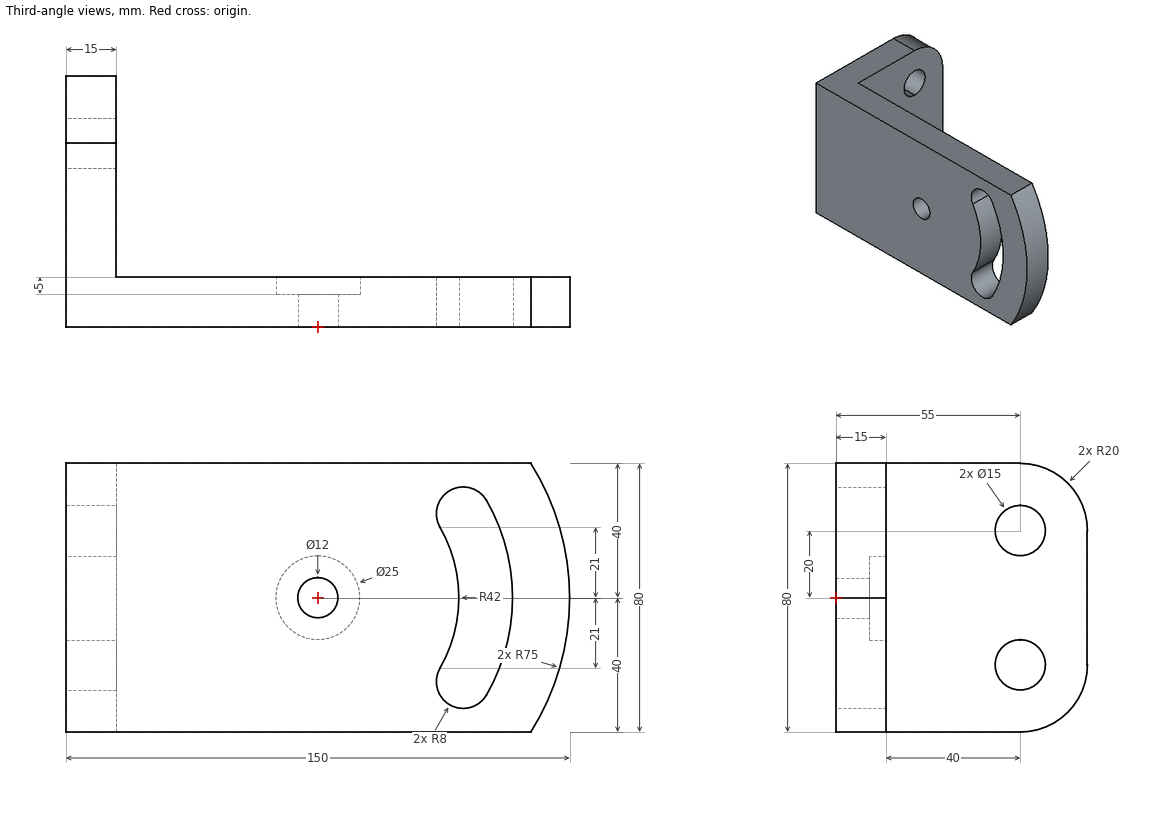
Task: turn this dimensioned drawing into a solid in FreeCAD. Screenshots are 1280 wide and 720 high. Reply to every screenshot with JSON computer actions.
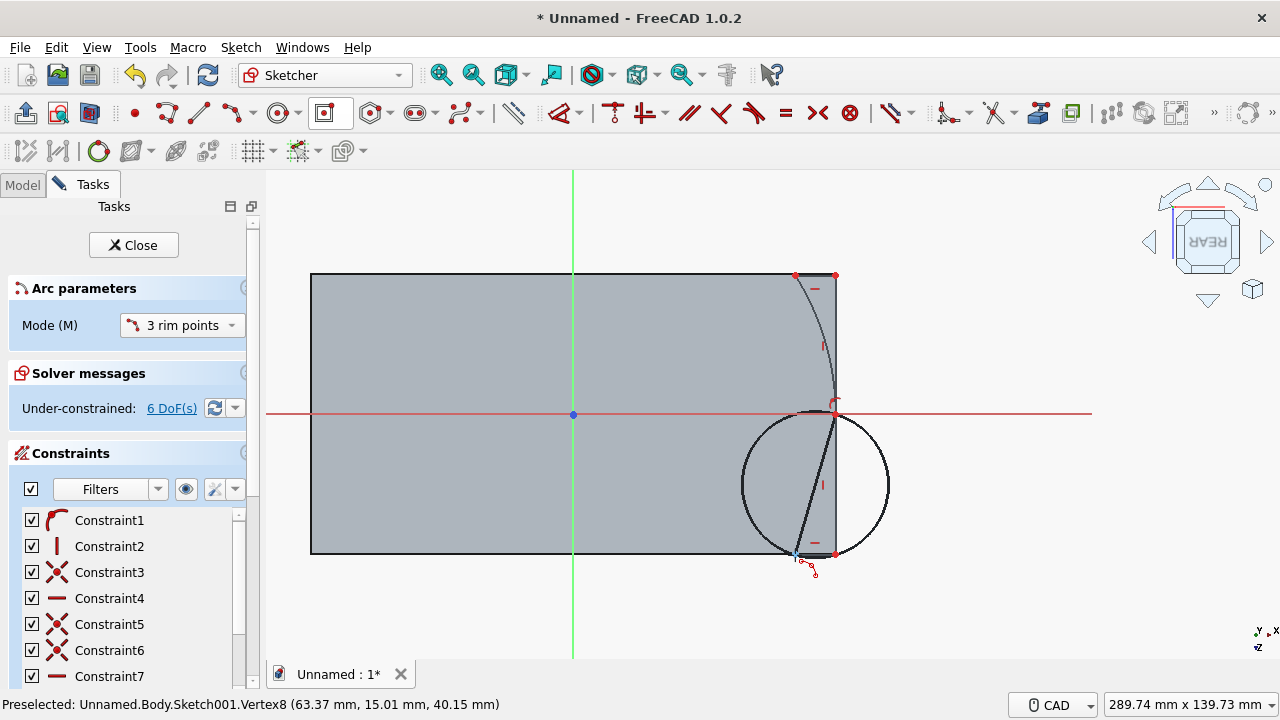
{"action": "scroll", "coordinate": [825, 487], "scroll_direction": "up", "scroll_amount": 3}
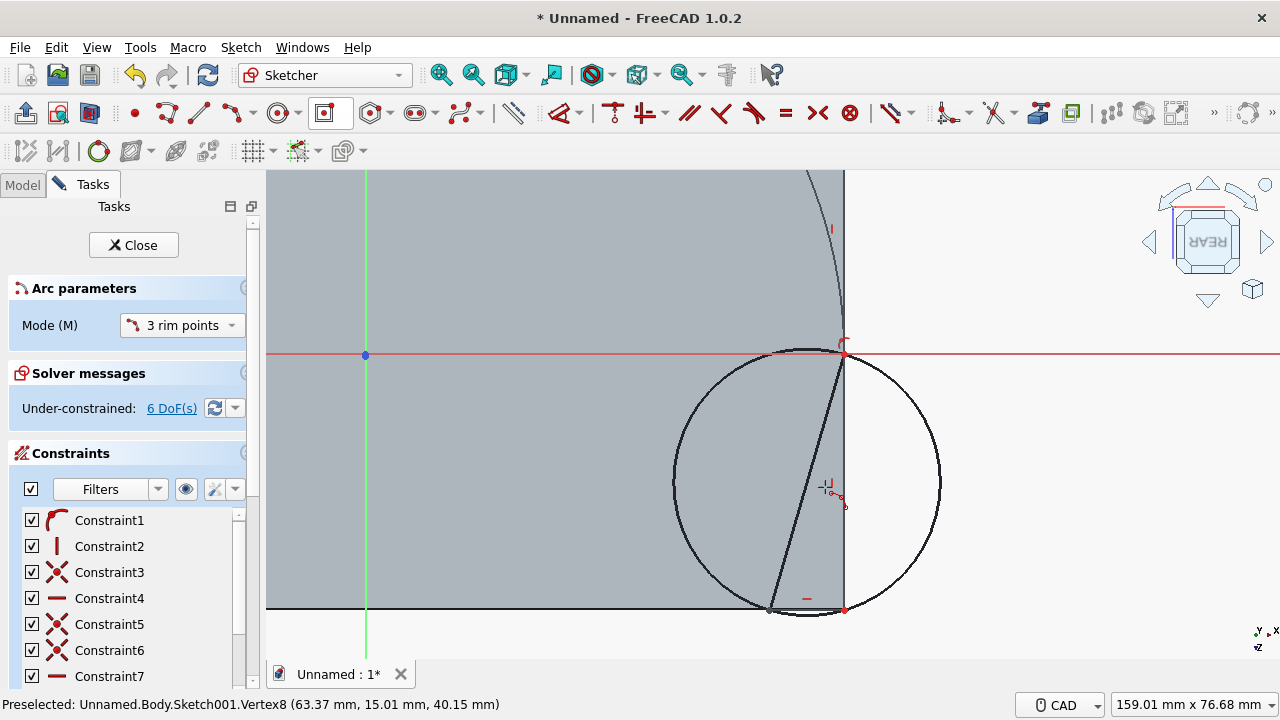
{"action": "left_click", "coordinate": [825, 487]}
{"action": "key", "text": "Escape"}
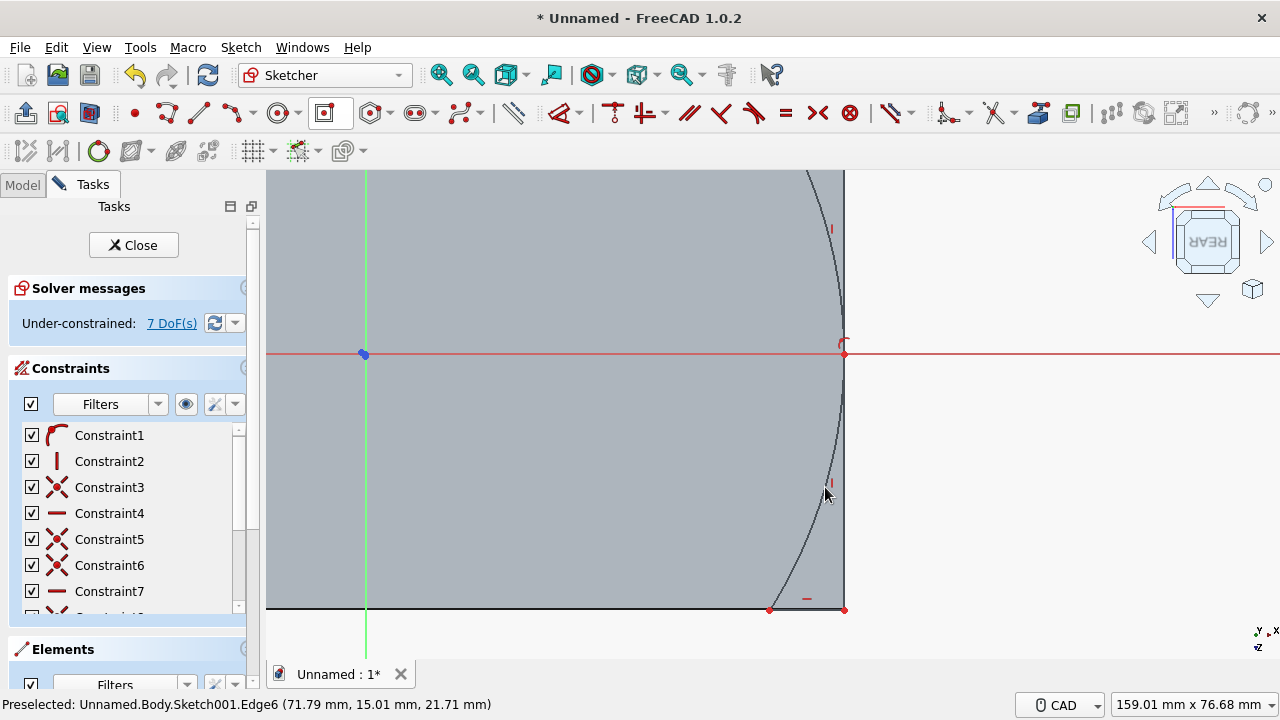
{"action": "left_click", "coordinate": [825, 223]}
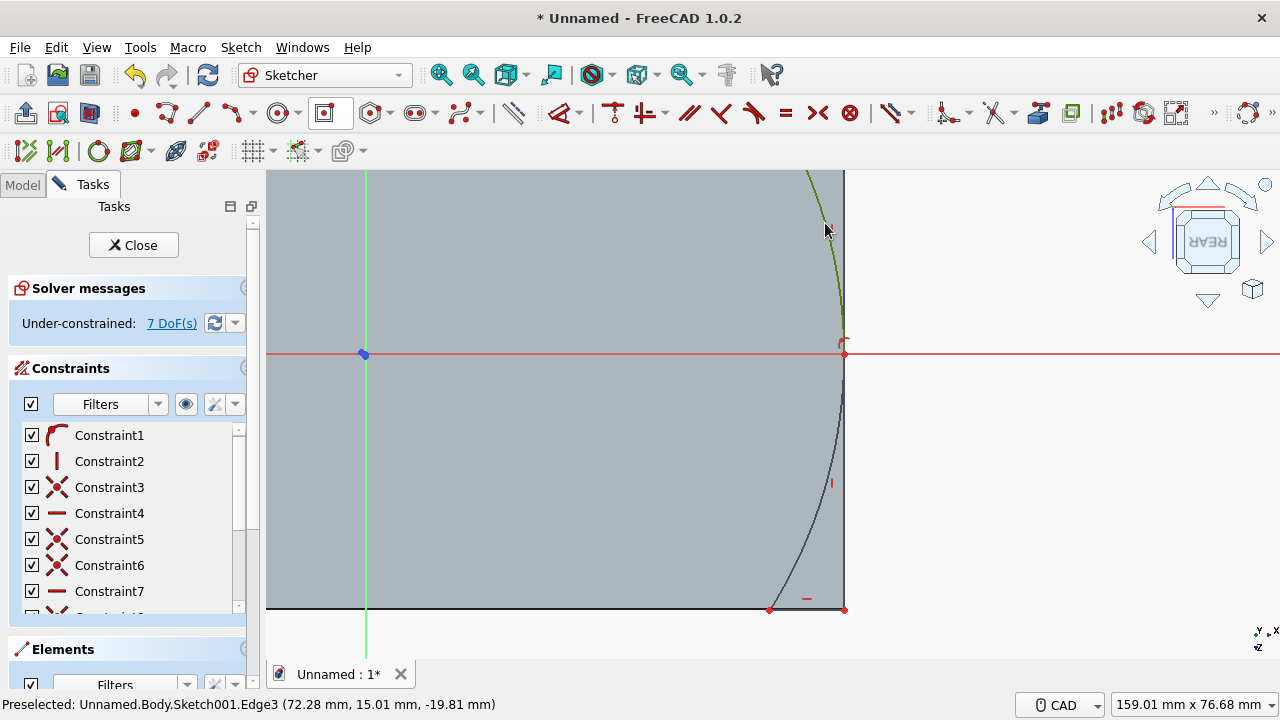
{"action": "left_click", "coordinate": [807, 539]}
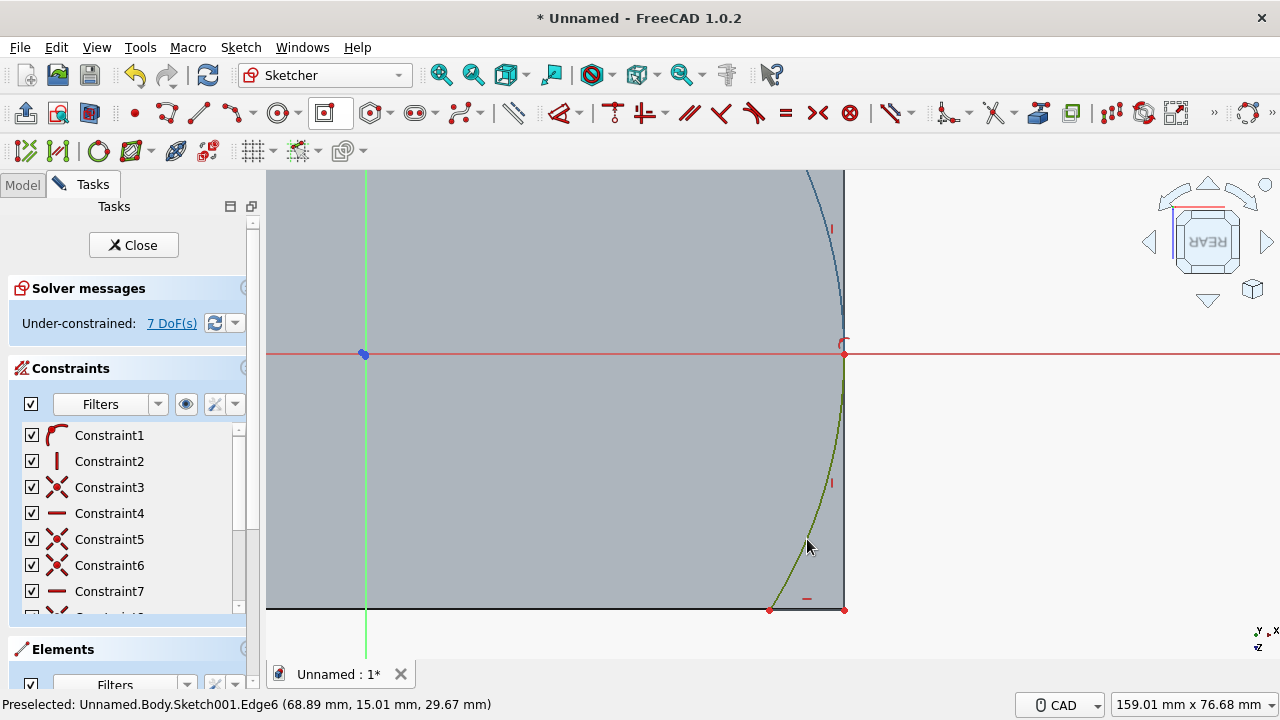
{"action": "left_click", "coordinate": [614, 114]}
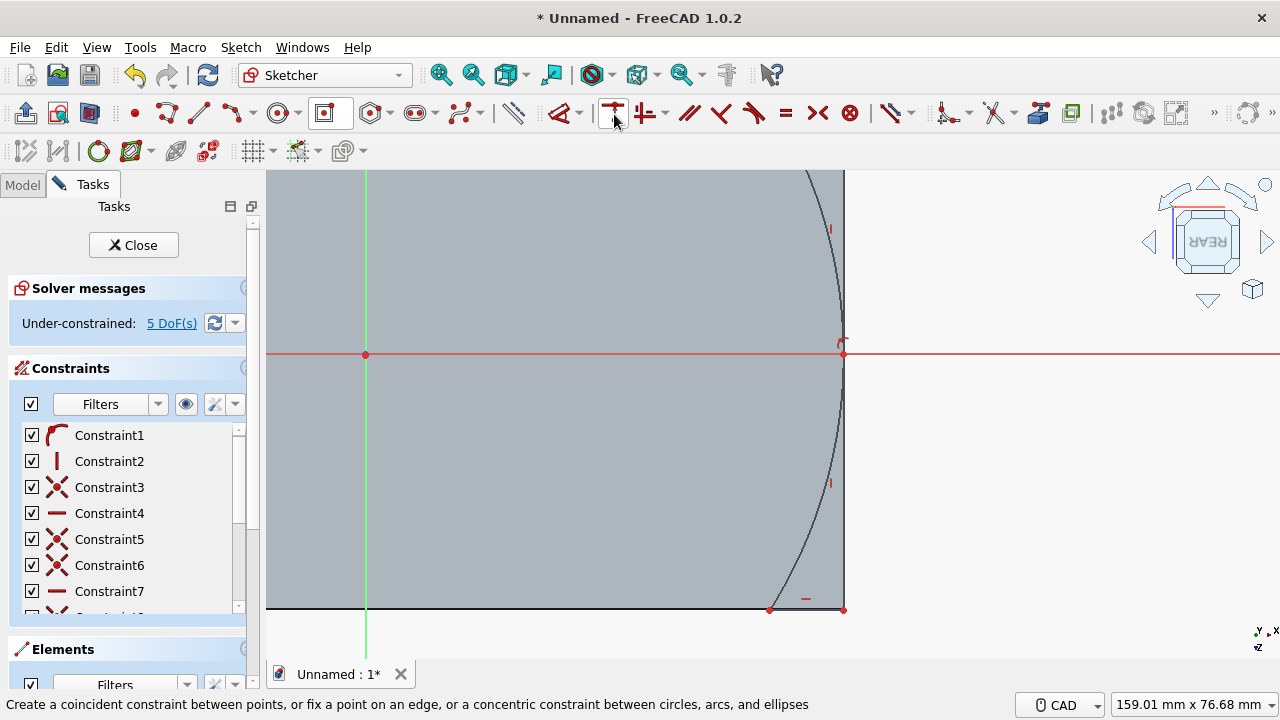
{"action": "left_click_drag", "start_coordinate": [356, 344], "coordinate": [376, 365]}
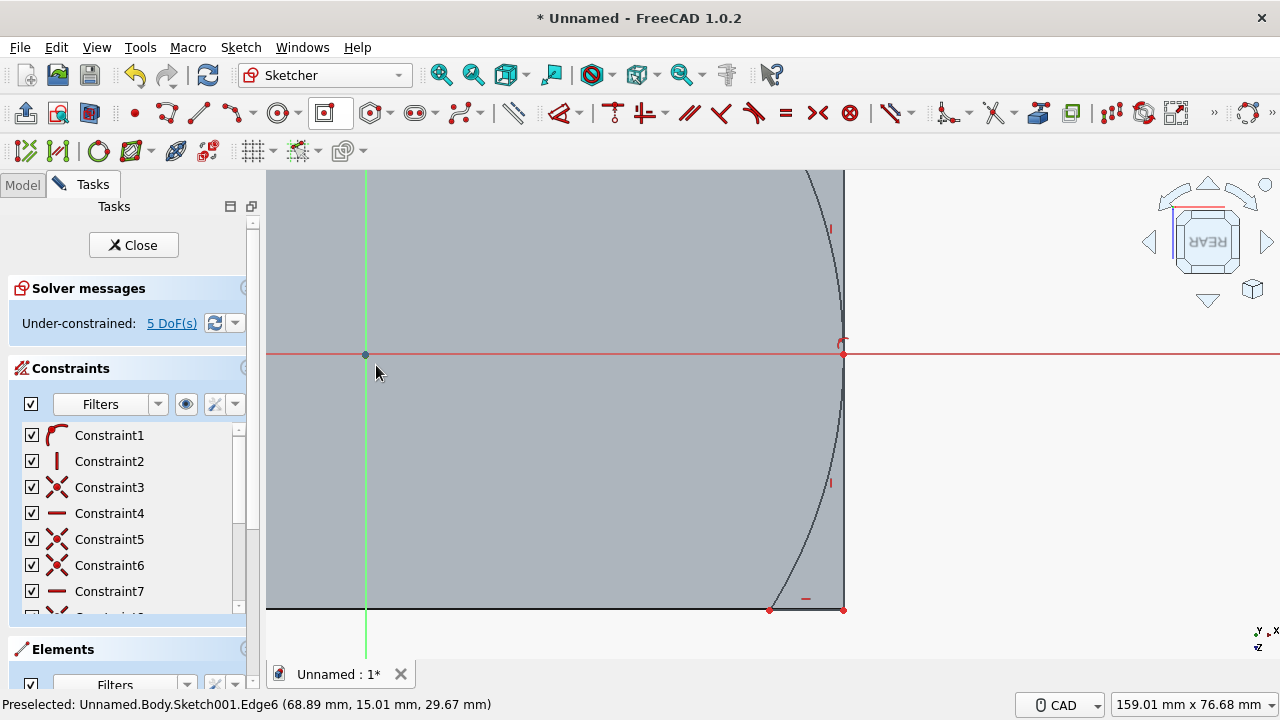
{"action": "left_click", "coordinate": [614, 114]}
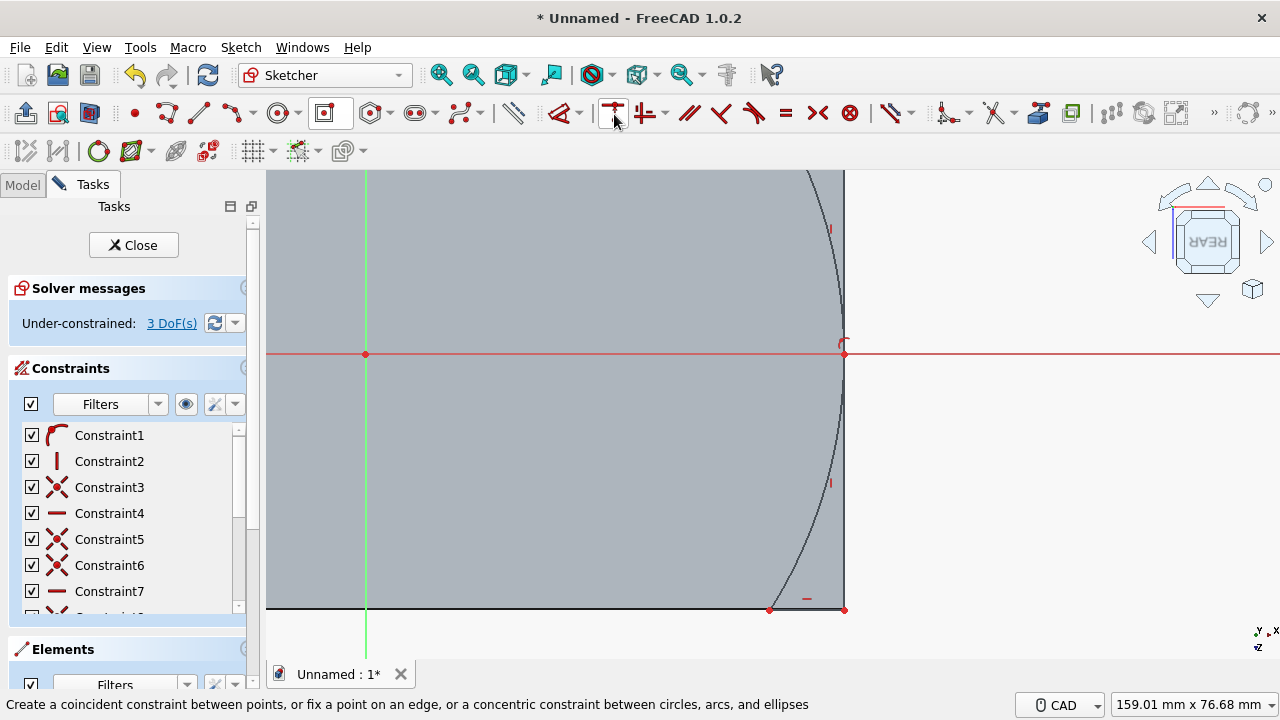
{"action": "left_click", "coordinate": [560, 114]}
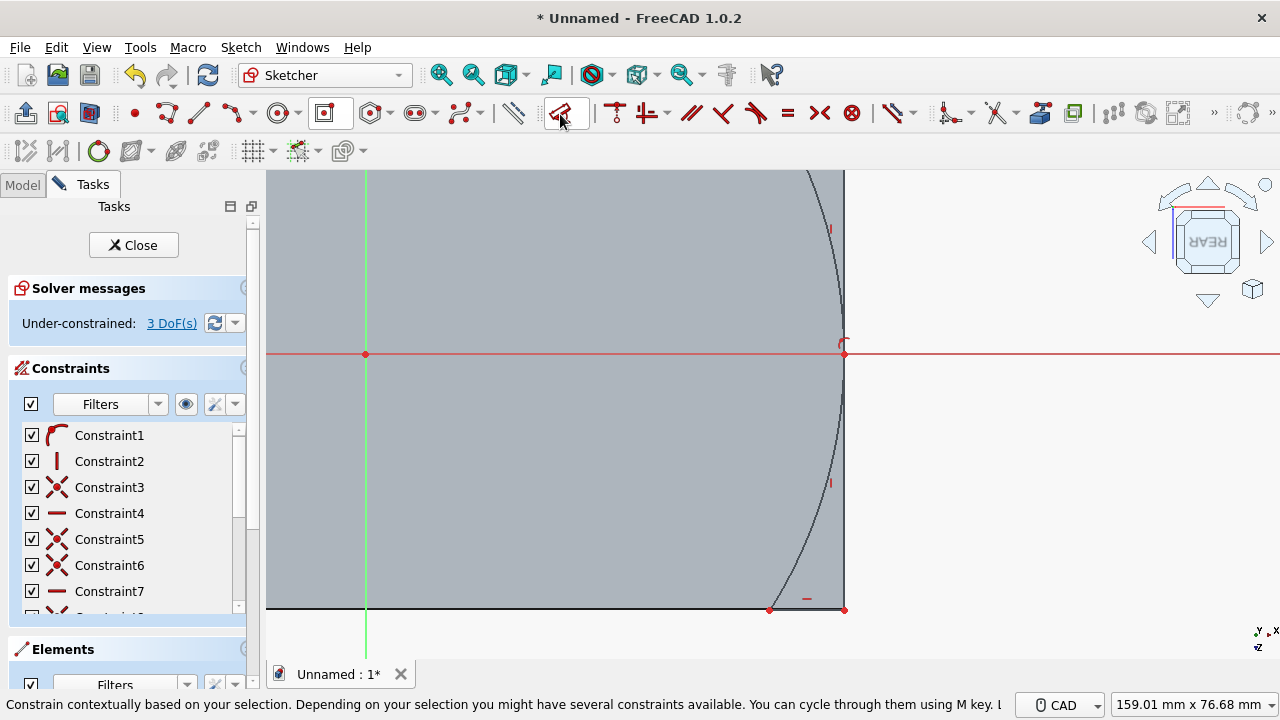
{"action": "left_click", "coordinate": [826, 223]}
{"action": "left_click", "coordinate": [864, 467]}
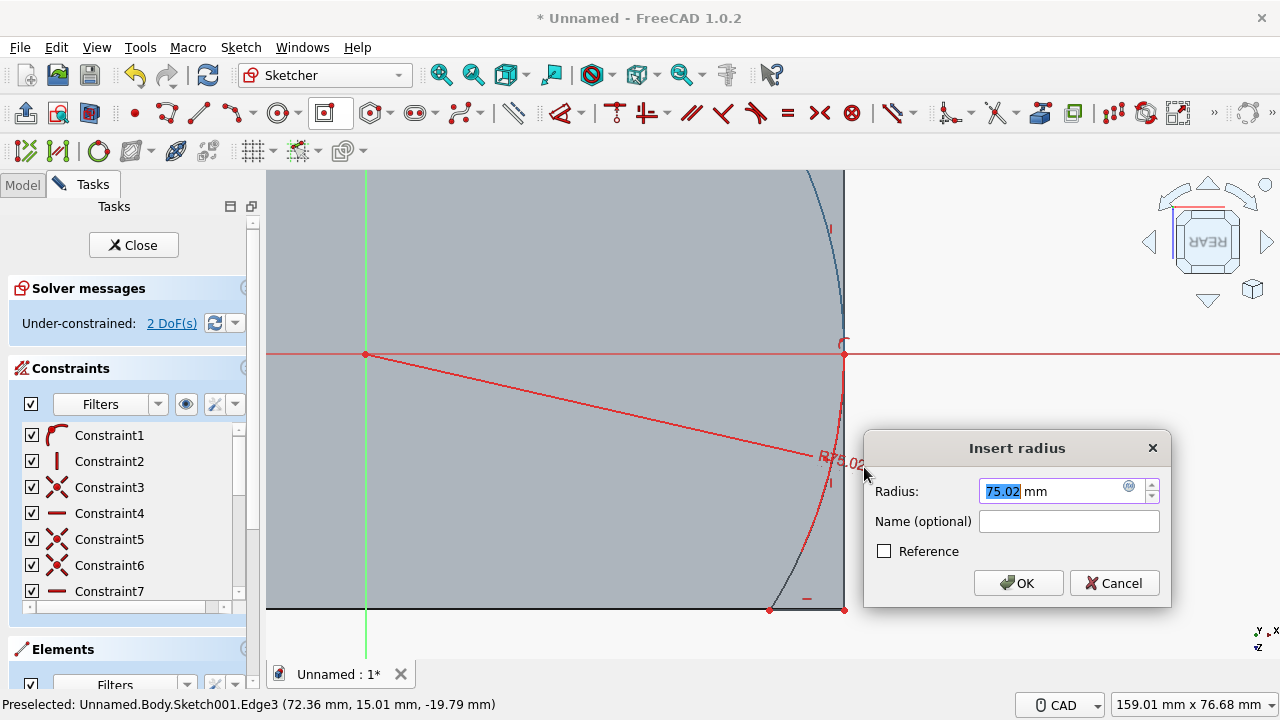
{"action": "type", "text": "75"}
{"action": "key", "text": "Return"}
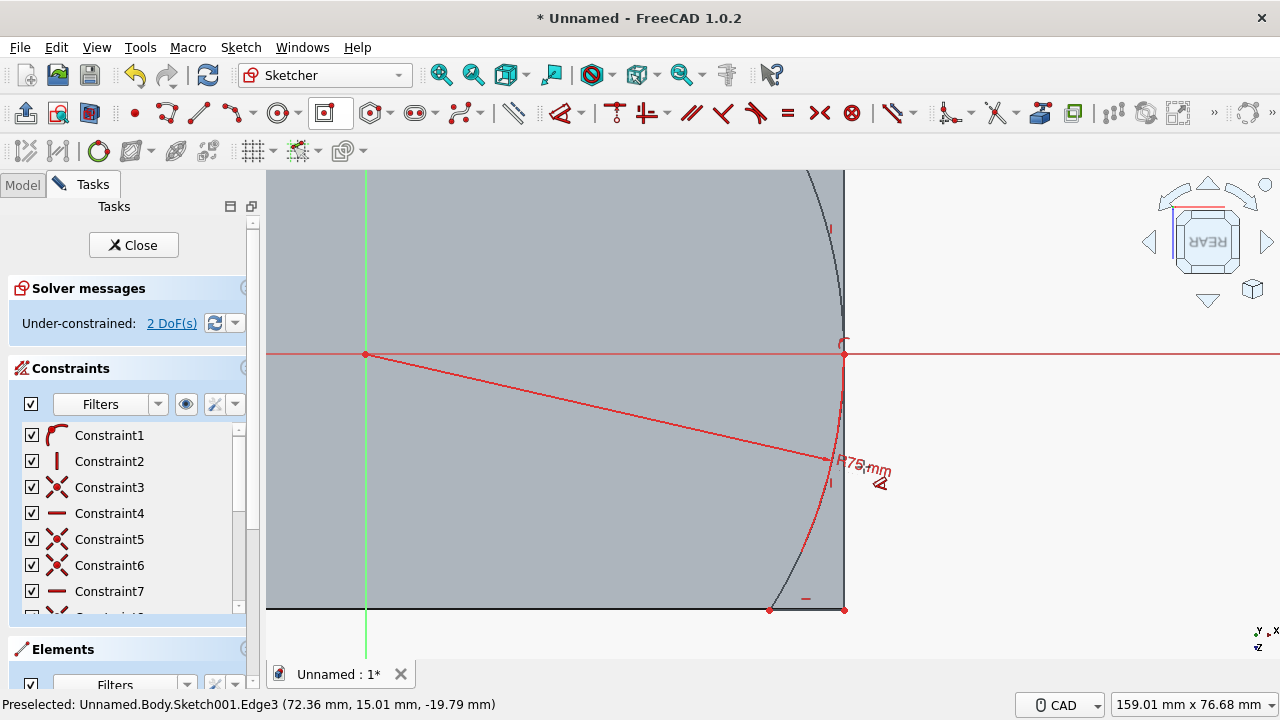
{"action": "scroll", "coordinate": [844, 253], "scroll_direction": "up", "scroll_amount": 2}